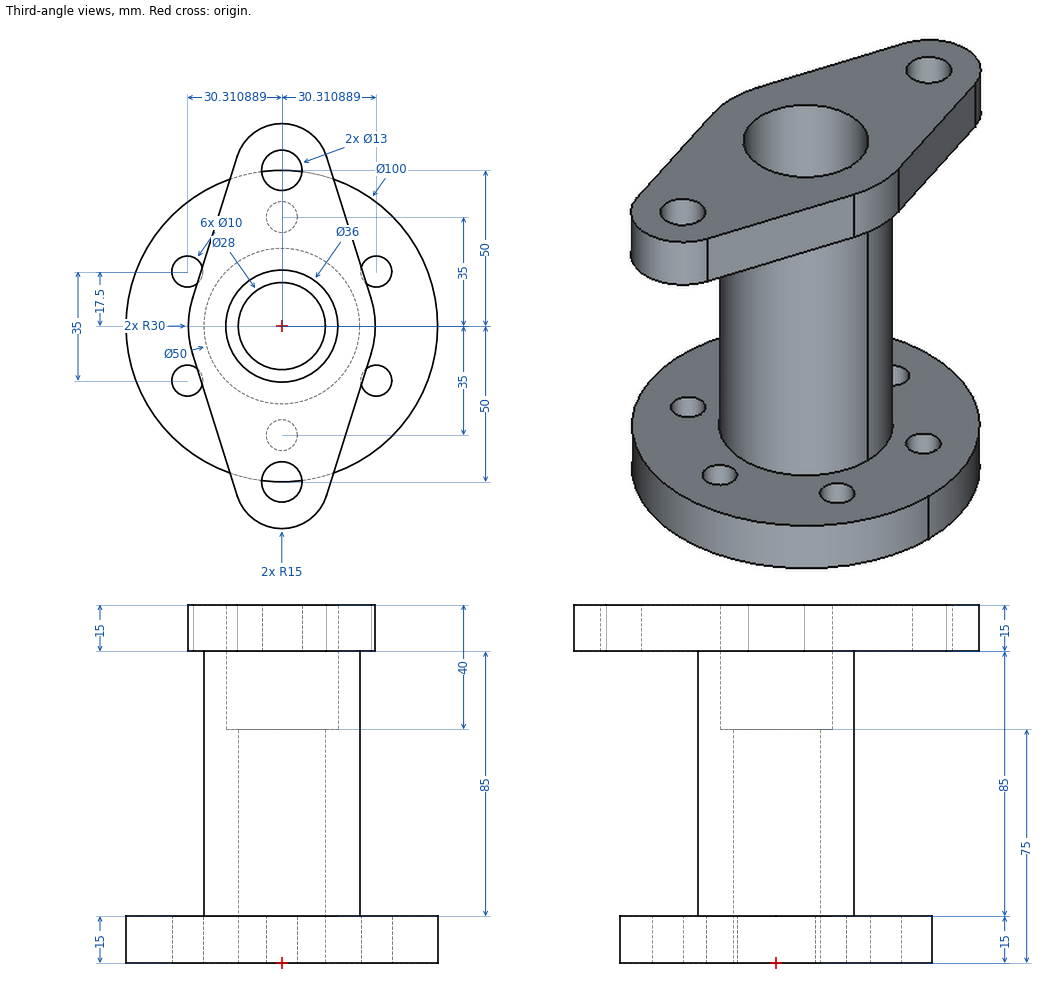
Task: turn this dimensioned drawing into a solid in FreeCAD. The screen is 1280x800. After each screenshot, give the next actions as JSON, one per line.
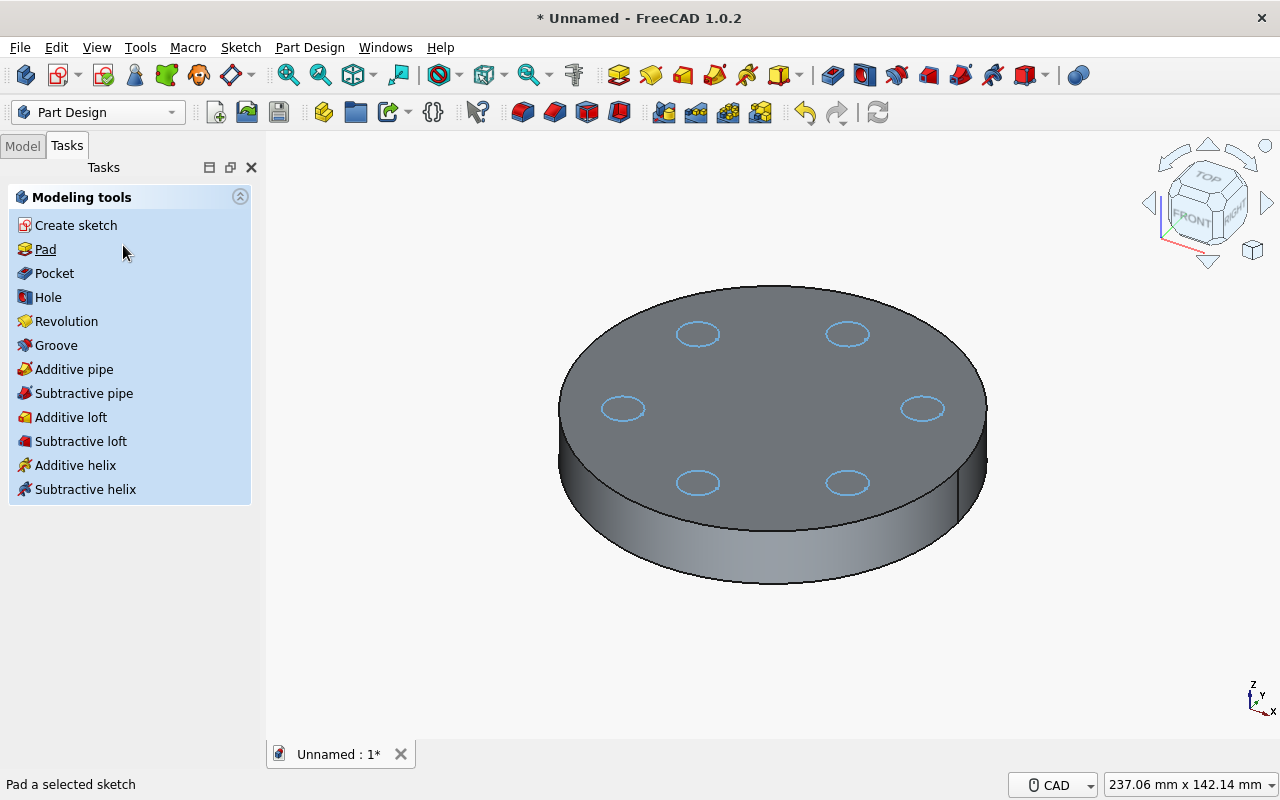
{"action": "left_click", "coordinate": [834, 76]}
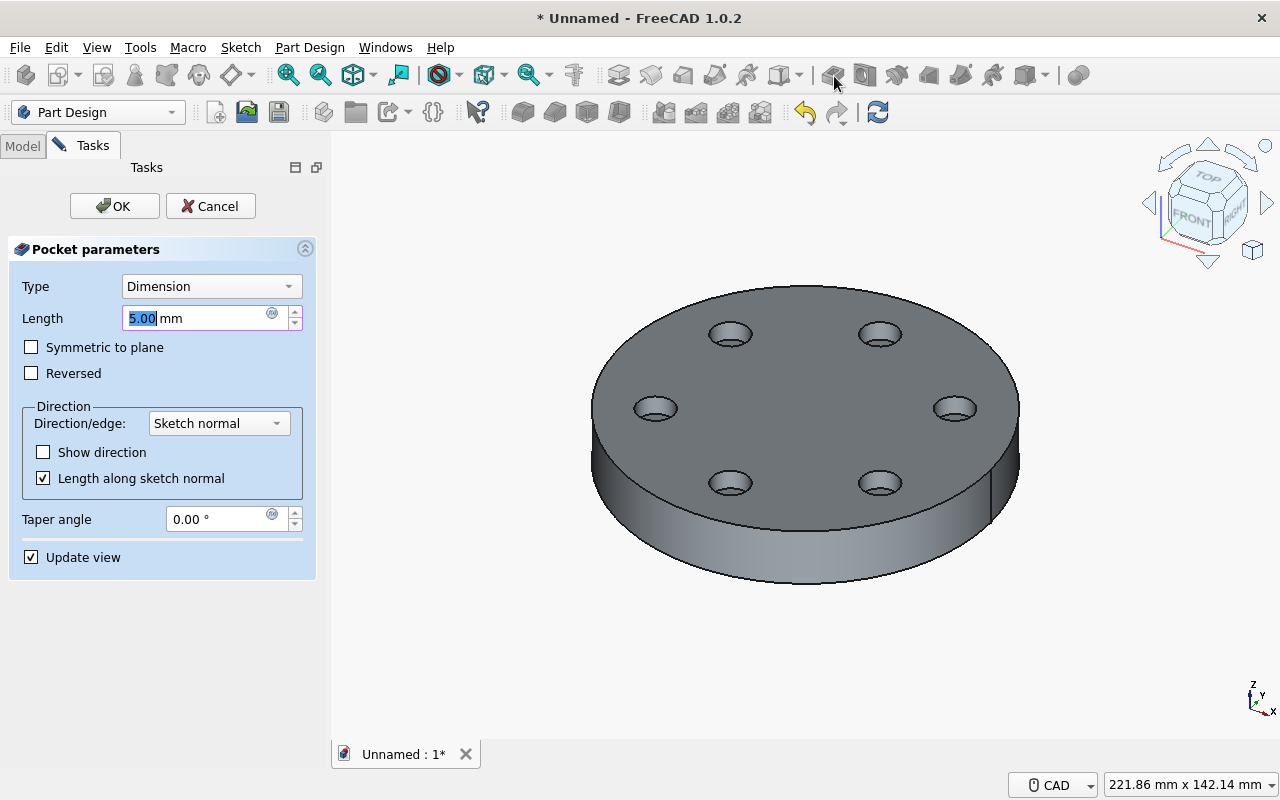
{"action": "type", "text": "15"}
{"action": "key", "text": "Tab"}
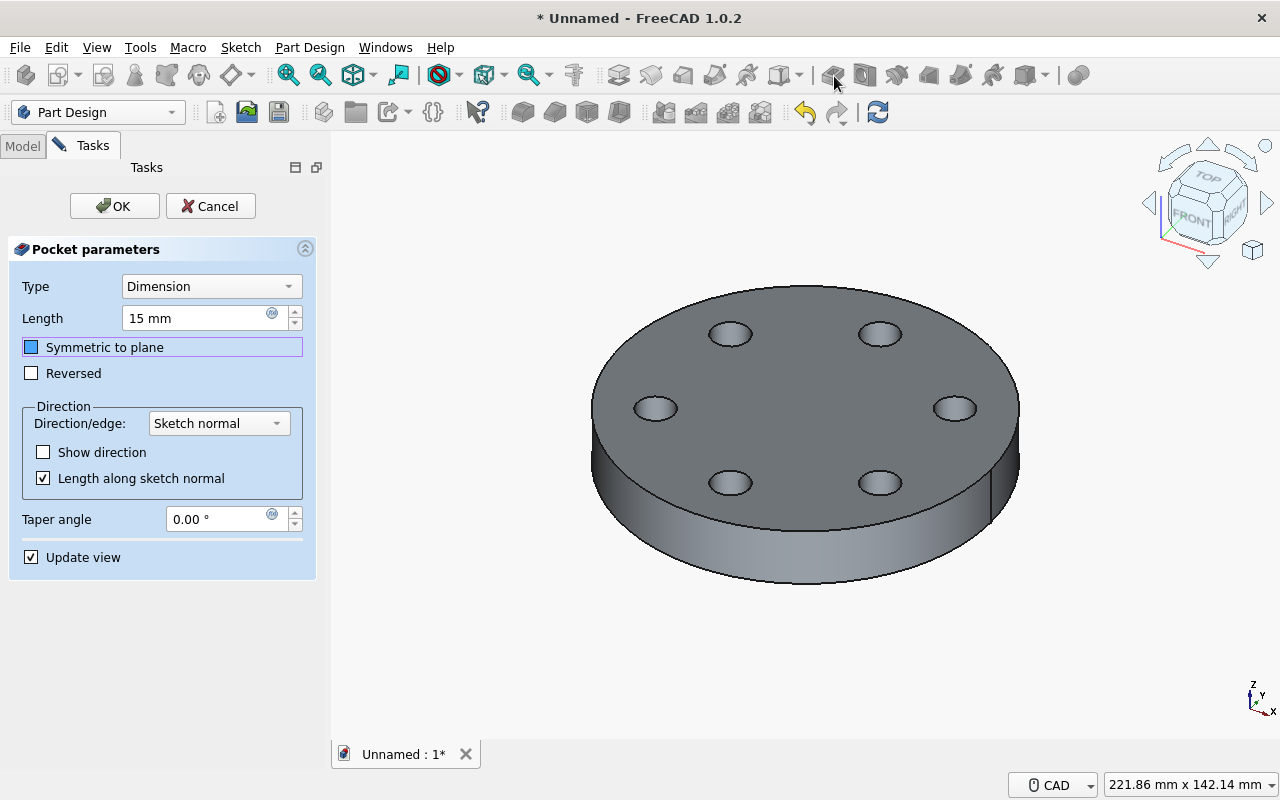
{"action": "left_click", "coordinate": [115, 206]}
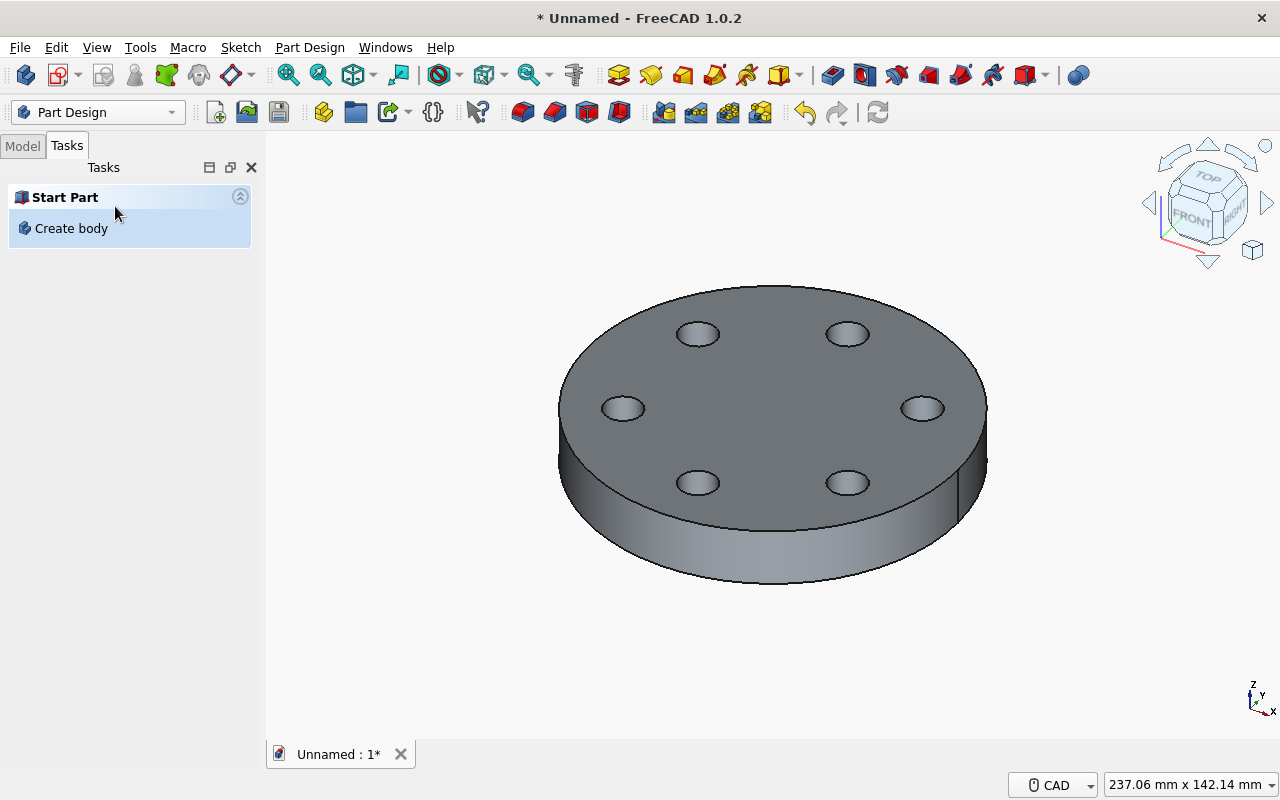
{"action": "left_click", "coordinate": [773, 408]}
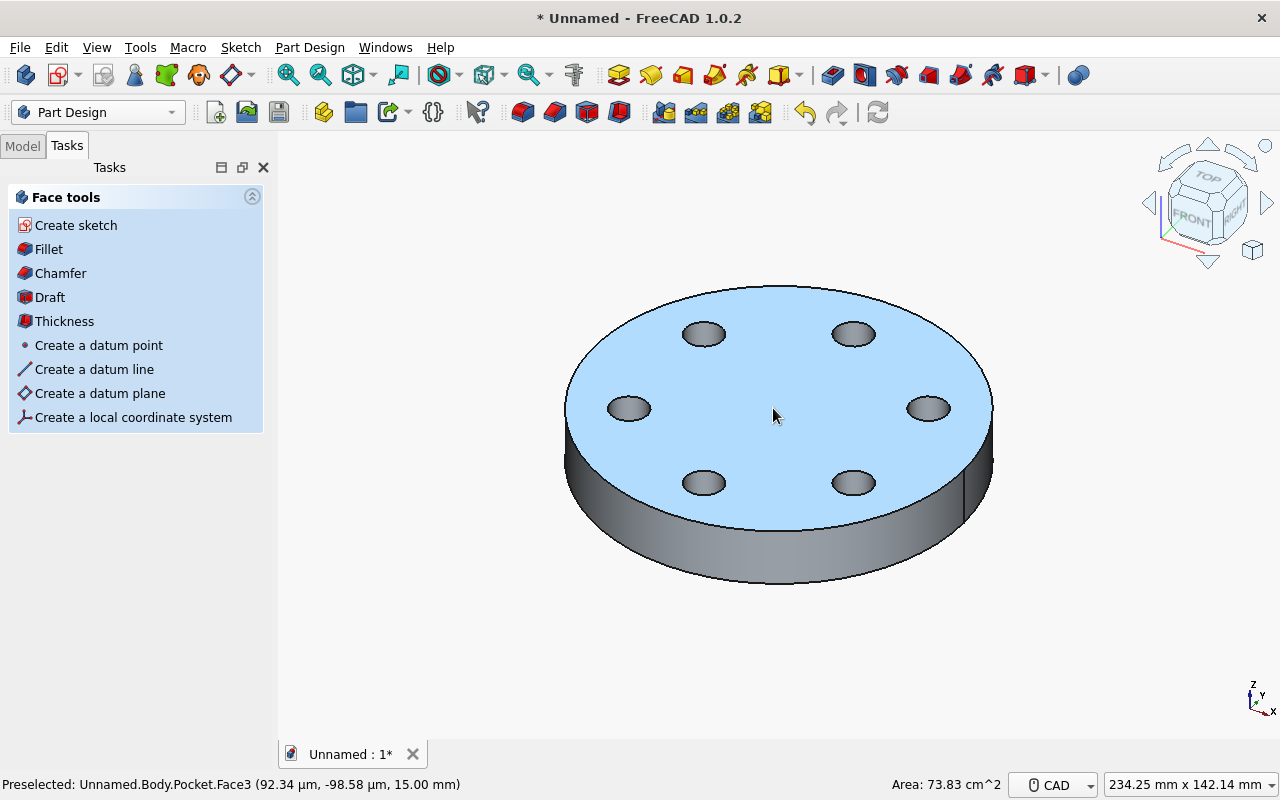
{"action": "left_click", "coordinate": [58, 76]}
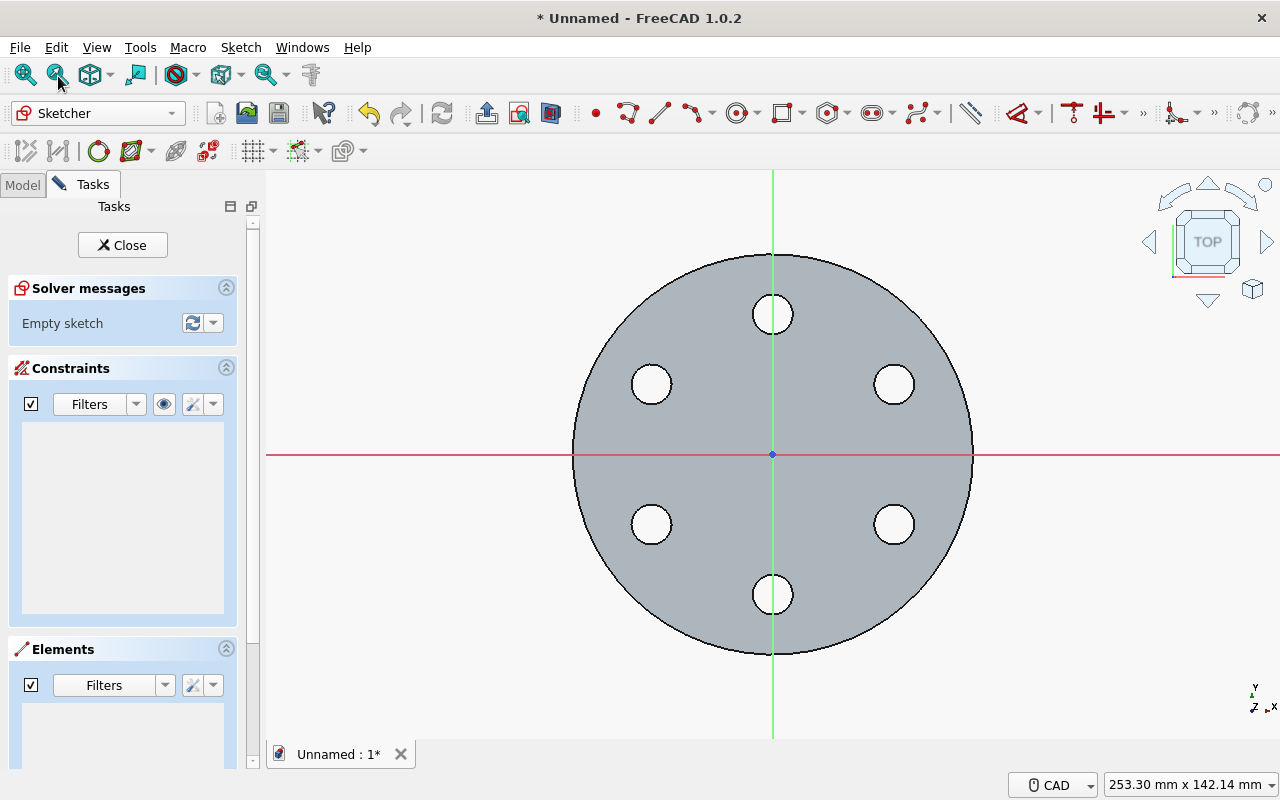
{"action": "scroll", "coordinate": [813, 454], "scroll_direction": "up", "scroll_amount": 5}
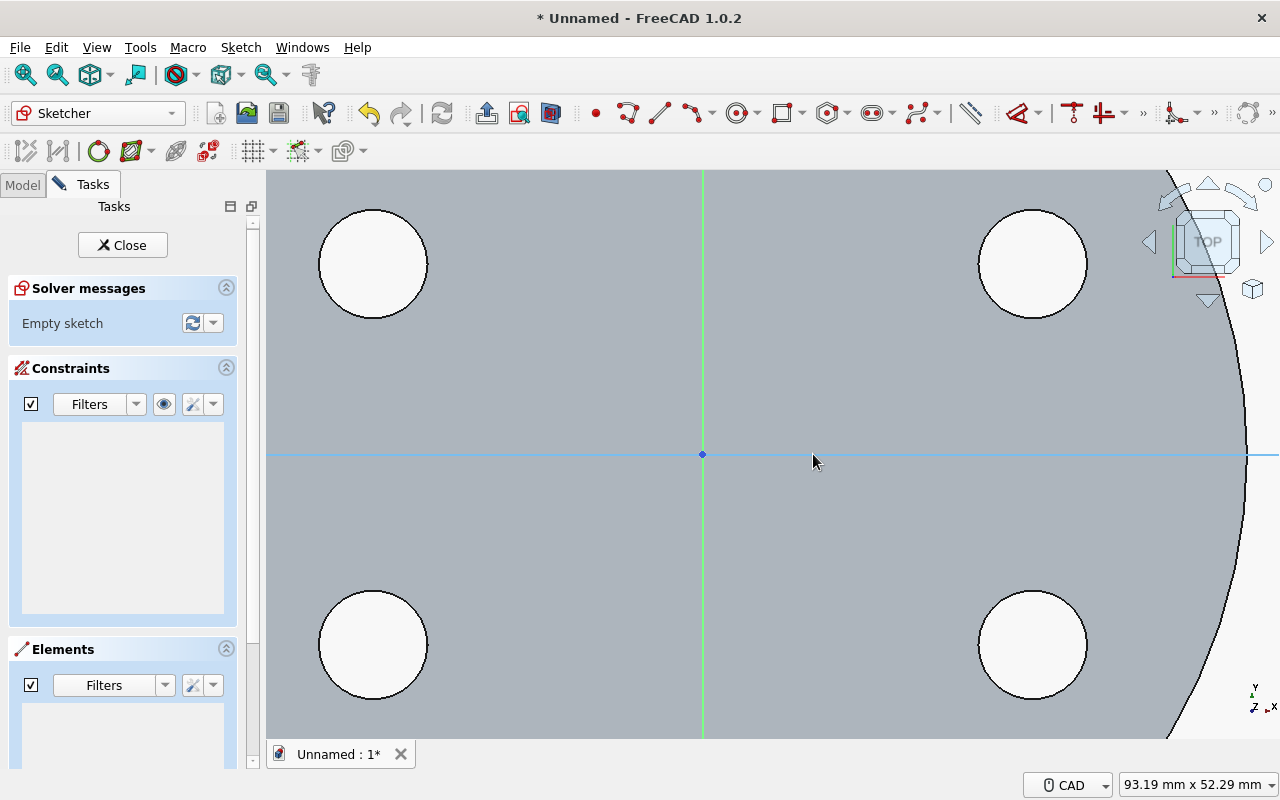
{"action": "left_click", "coordinate": [738, 114]}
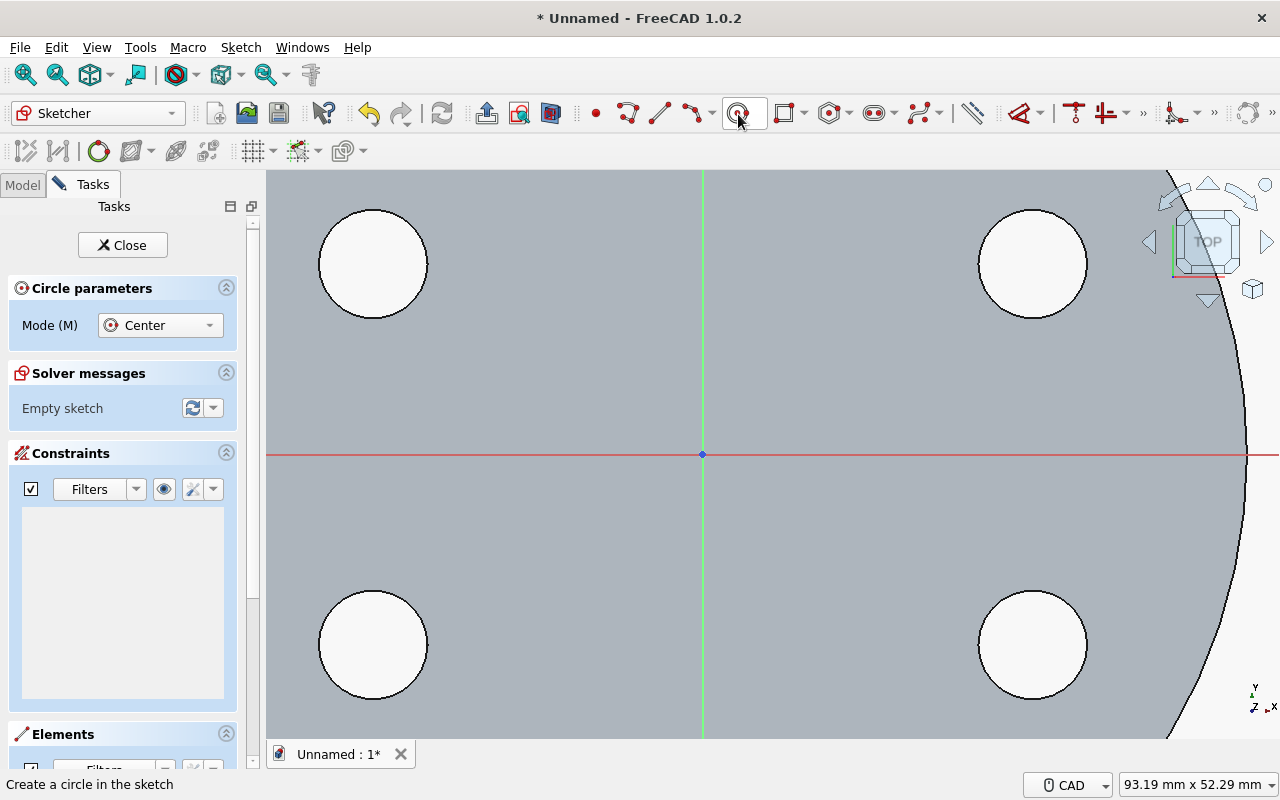
{"action": "left_click", "coordinate": [703, 454]}
{"action": "mouse_move", "coordinate": [841, 316]}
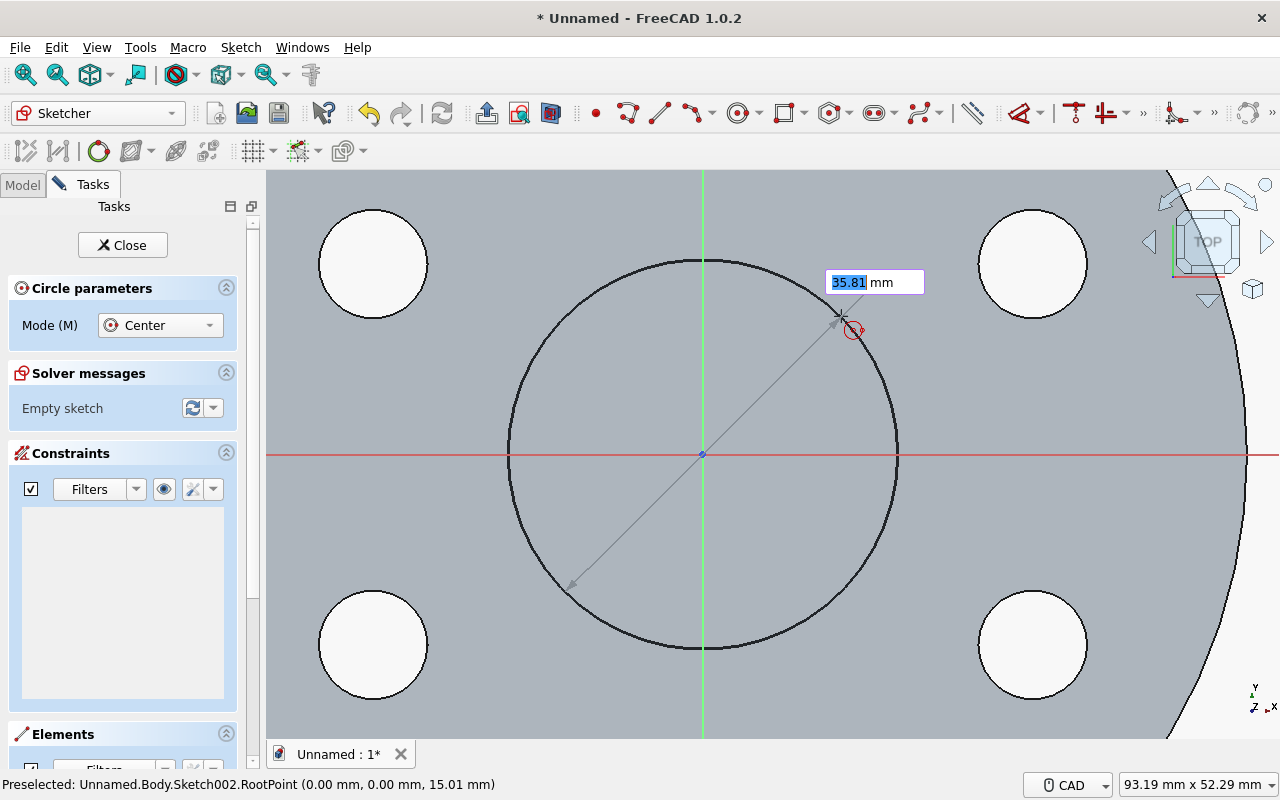
{"action": "type", "text": "36"}
{"action": "key", "text": "Return"}
{"action": "key", "text": "Escape"}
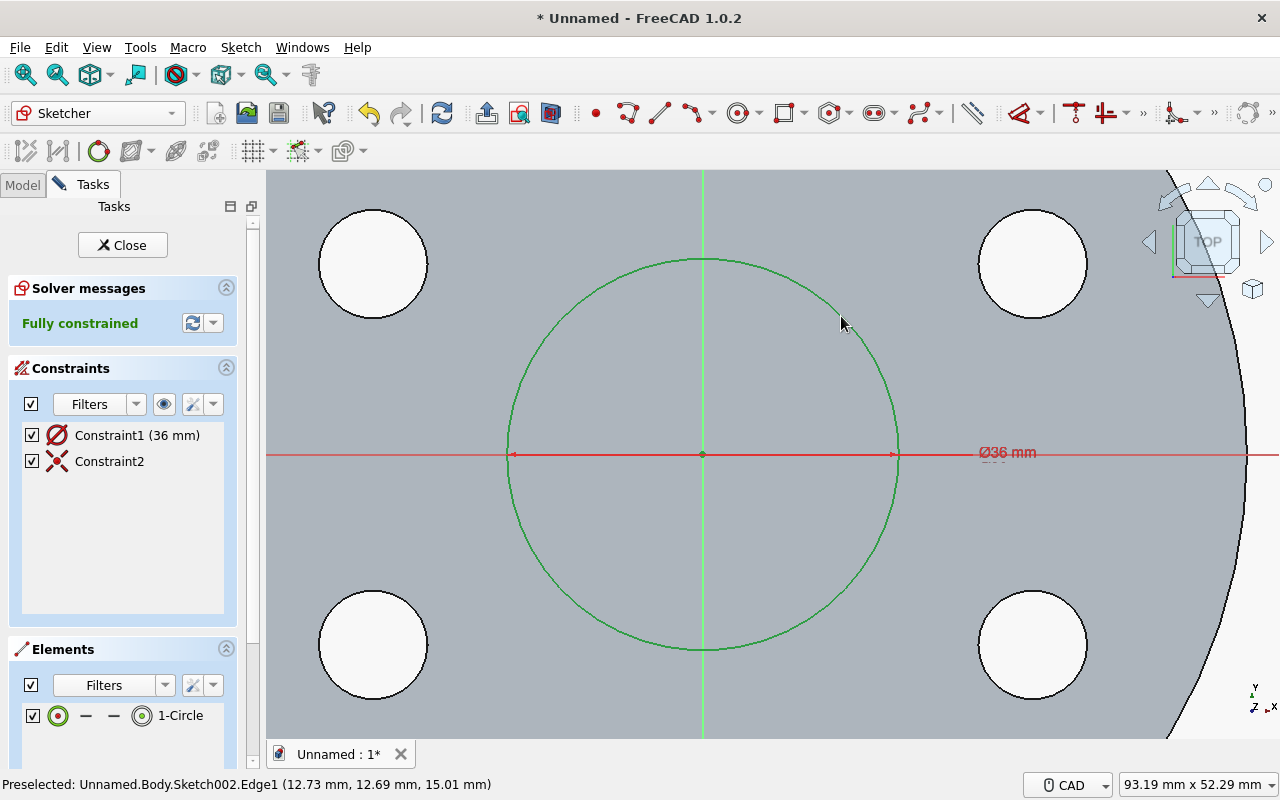
{"action": "left_click", "coordinate": [123, 245]}